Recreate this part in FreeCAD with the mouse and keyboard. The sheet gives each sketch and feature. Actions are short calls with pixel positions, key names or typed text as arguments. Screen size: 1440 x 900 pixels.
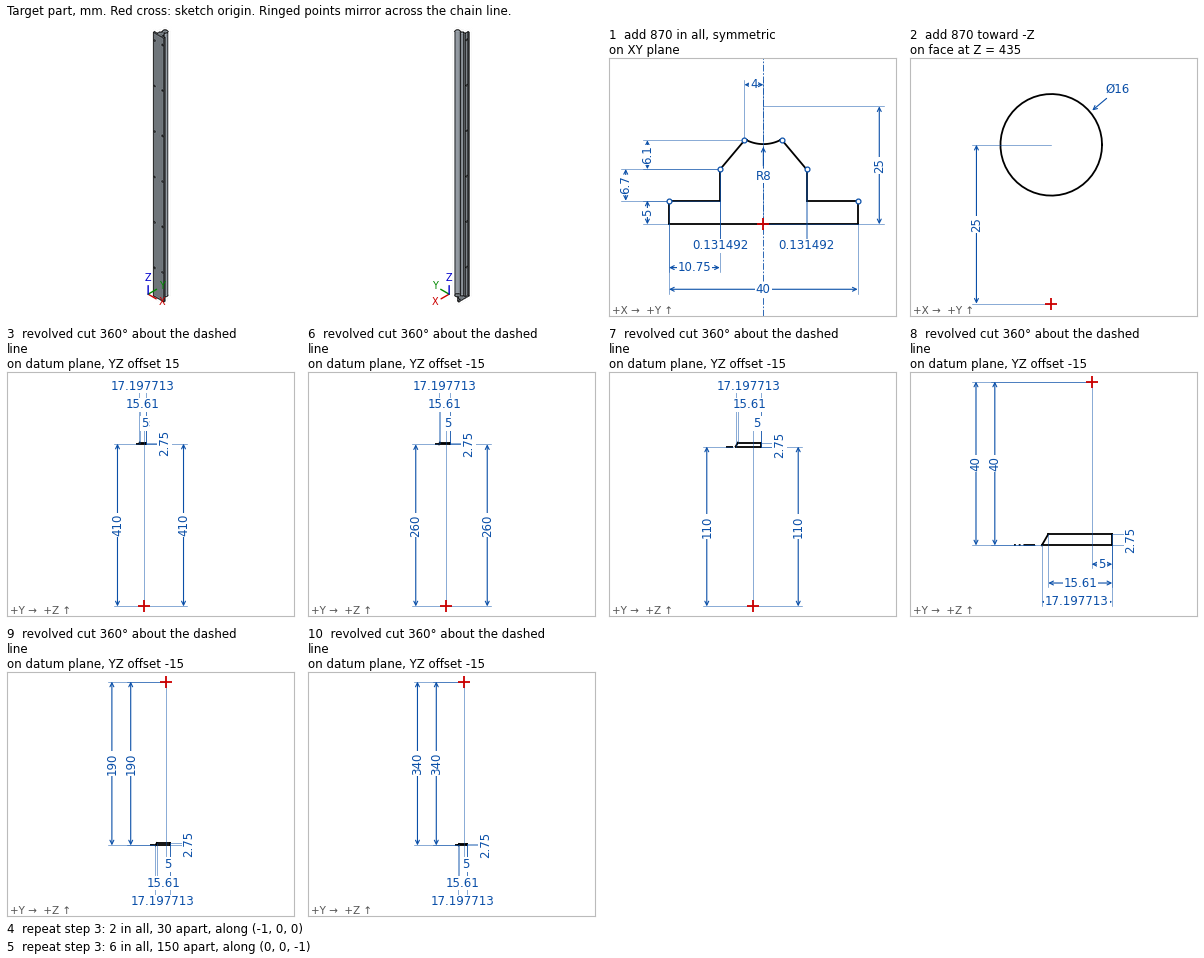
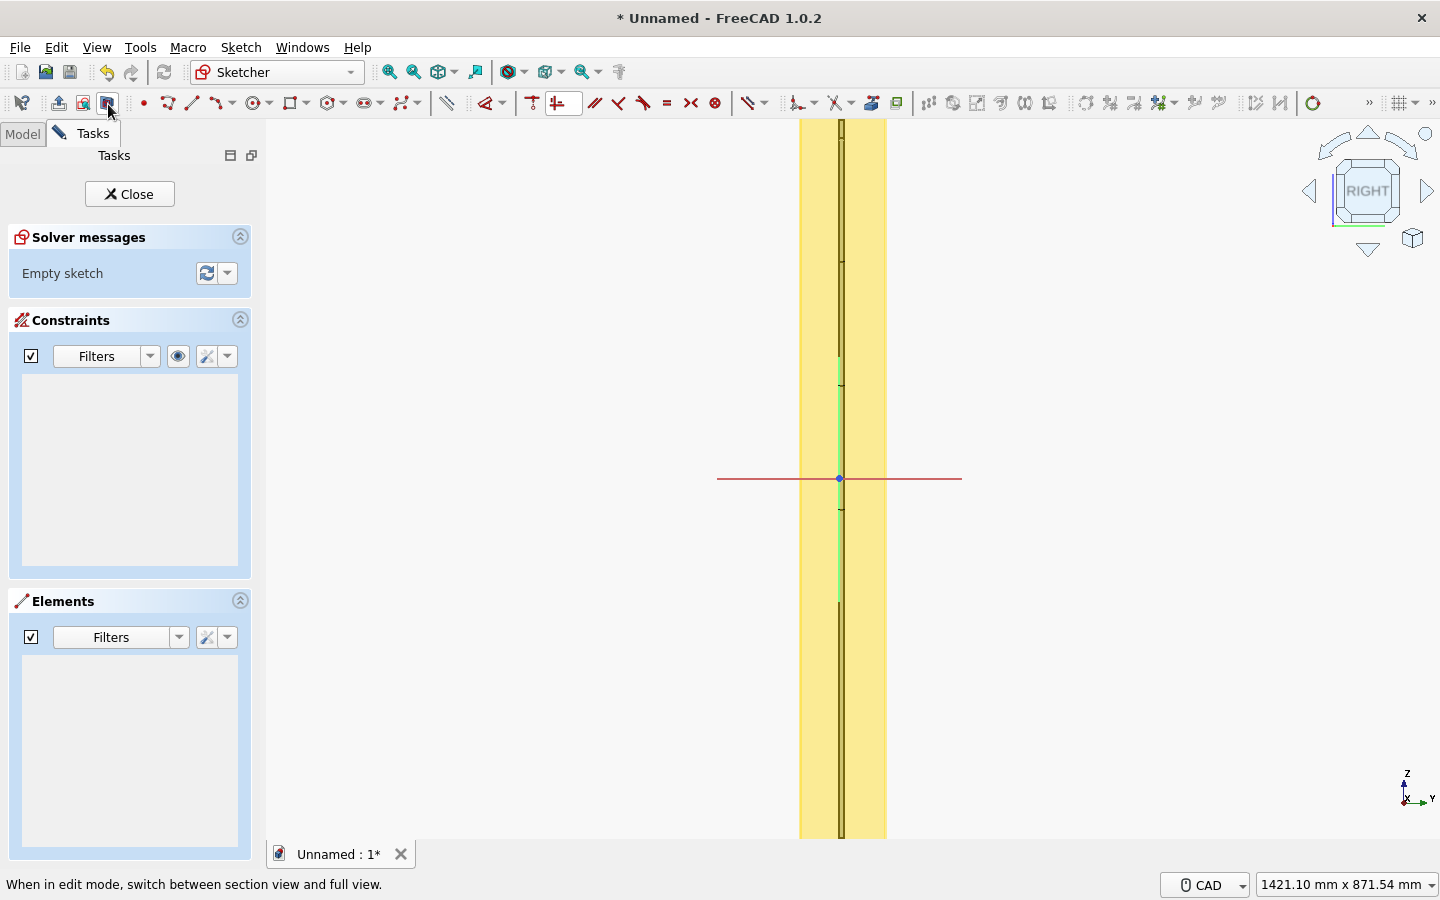
scroll(836, 643, up, 15)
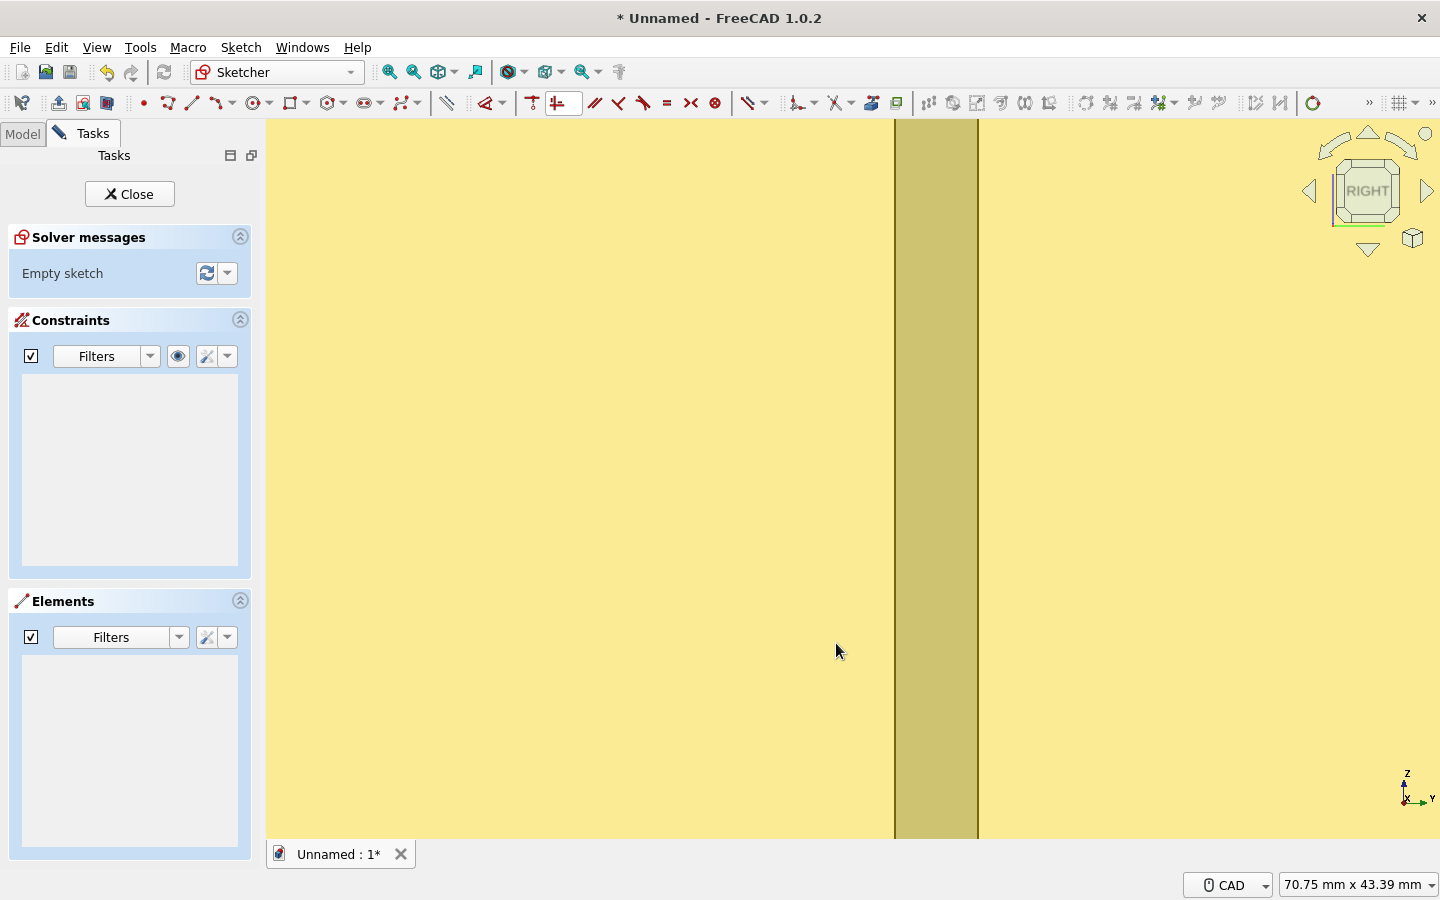
scroll(770, 448, up, 3)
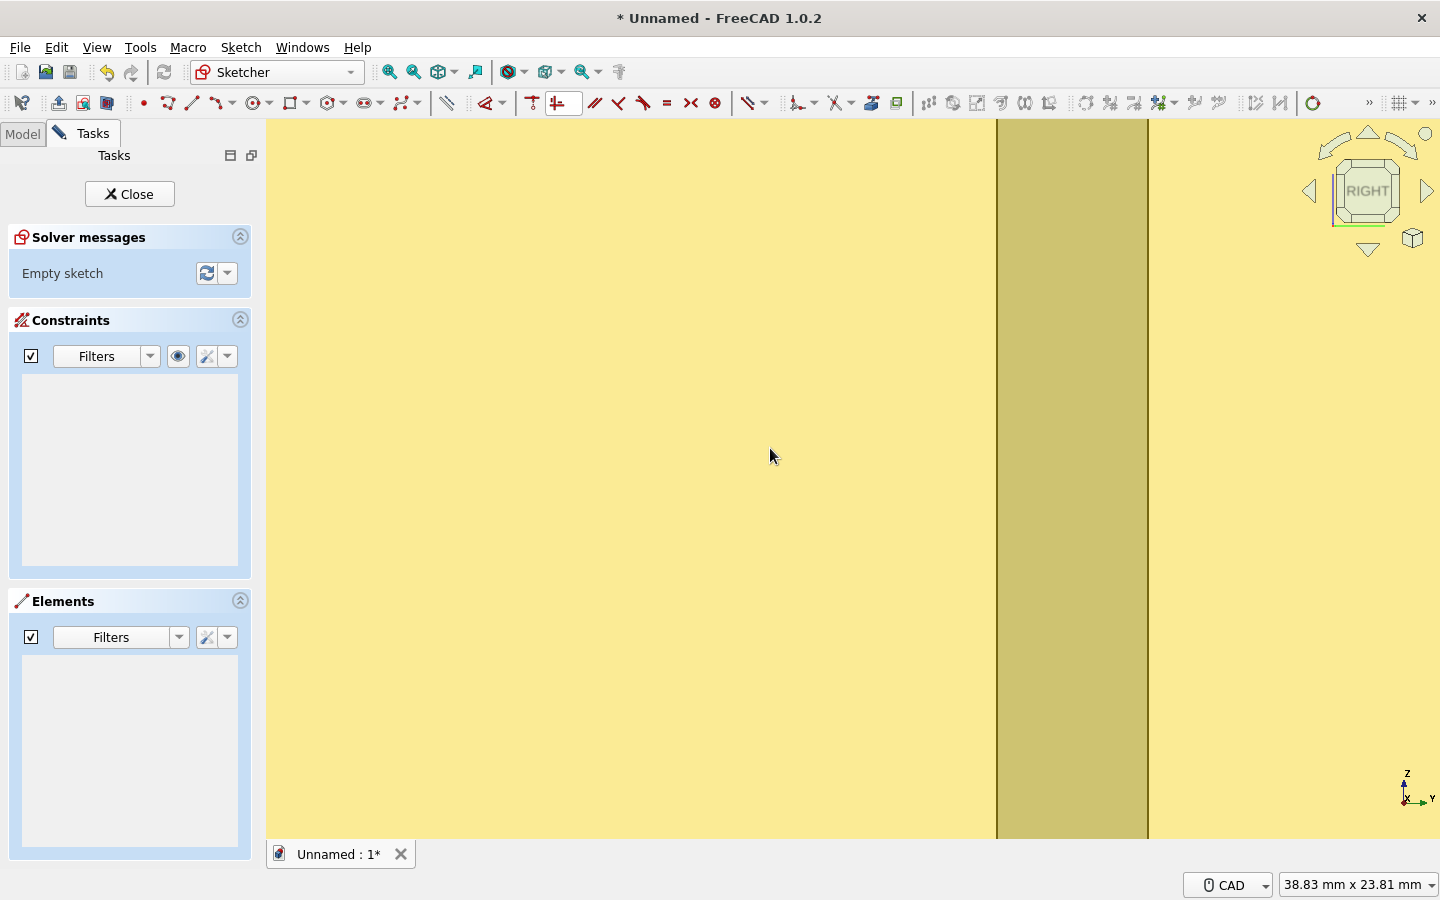
click(168, 104)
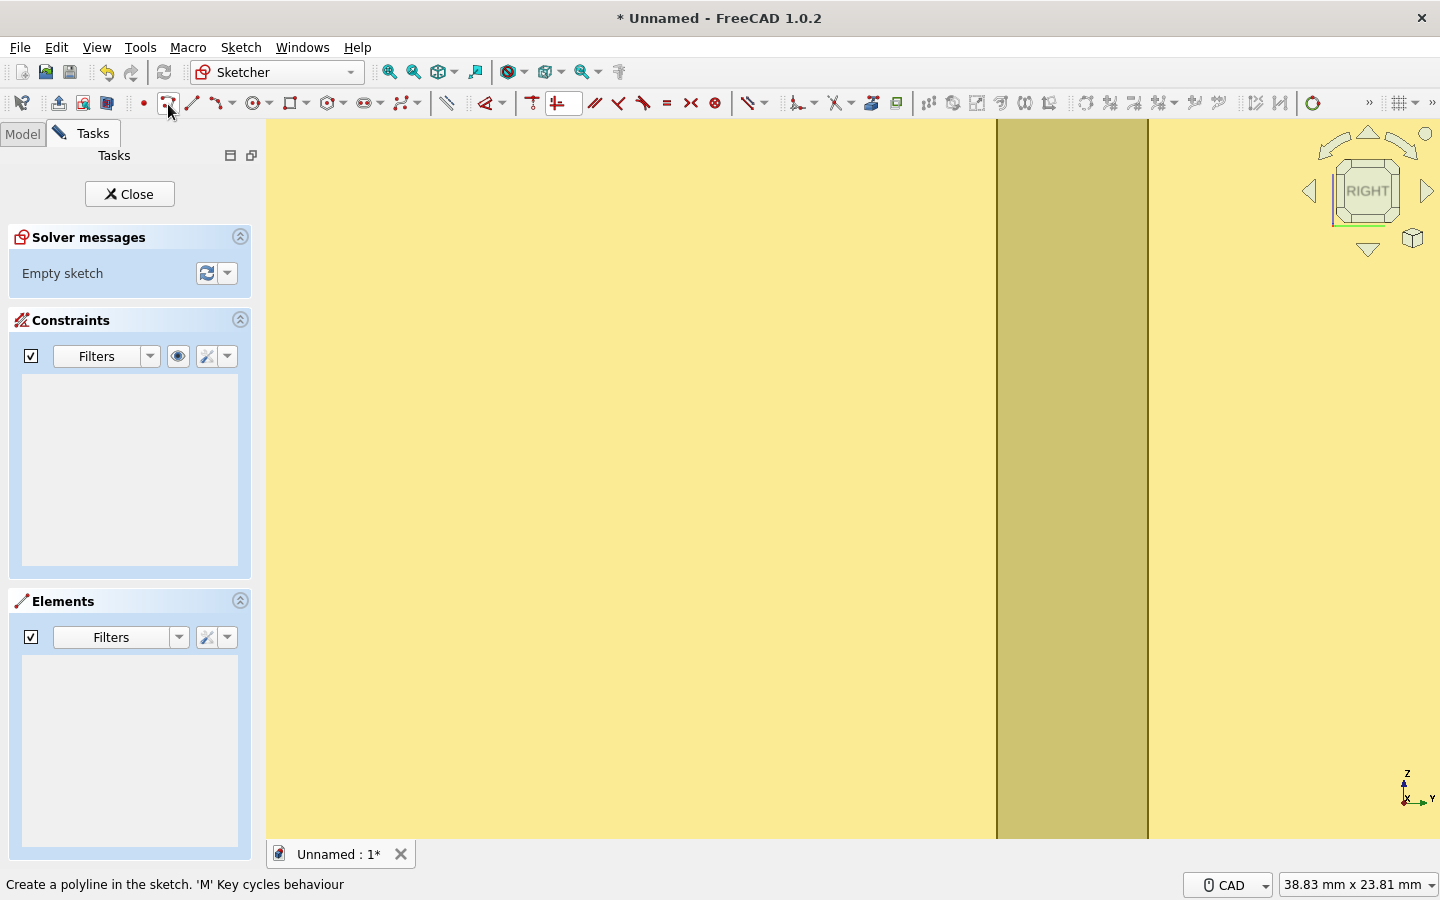
click(1148, 437)
click(676, 437)
click(628, 520)
click(1148, 520)
click(1148, 438)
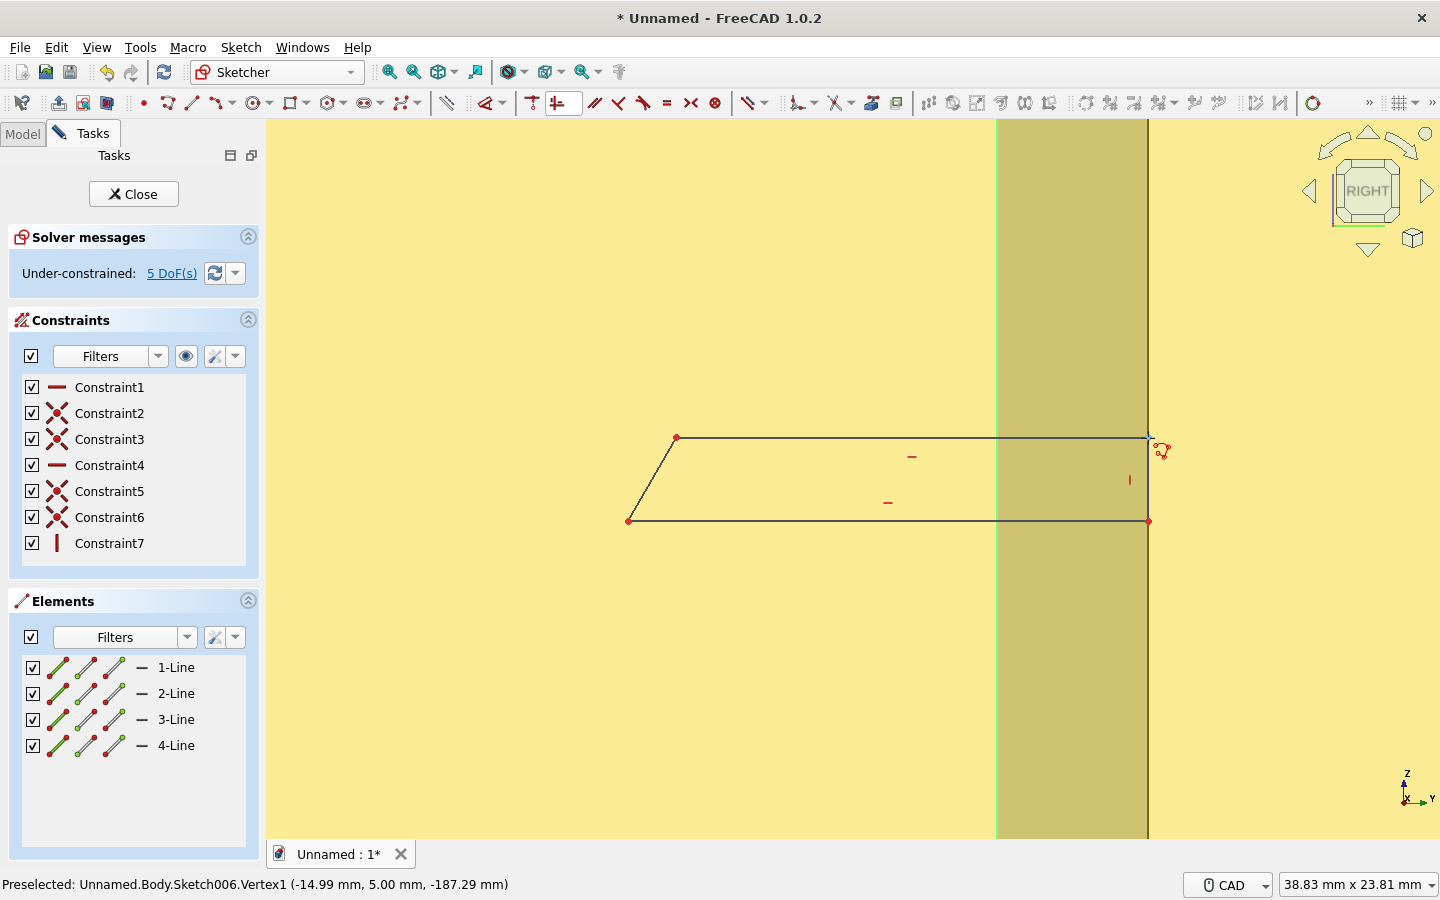
click(192, 104)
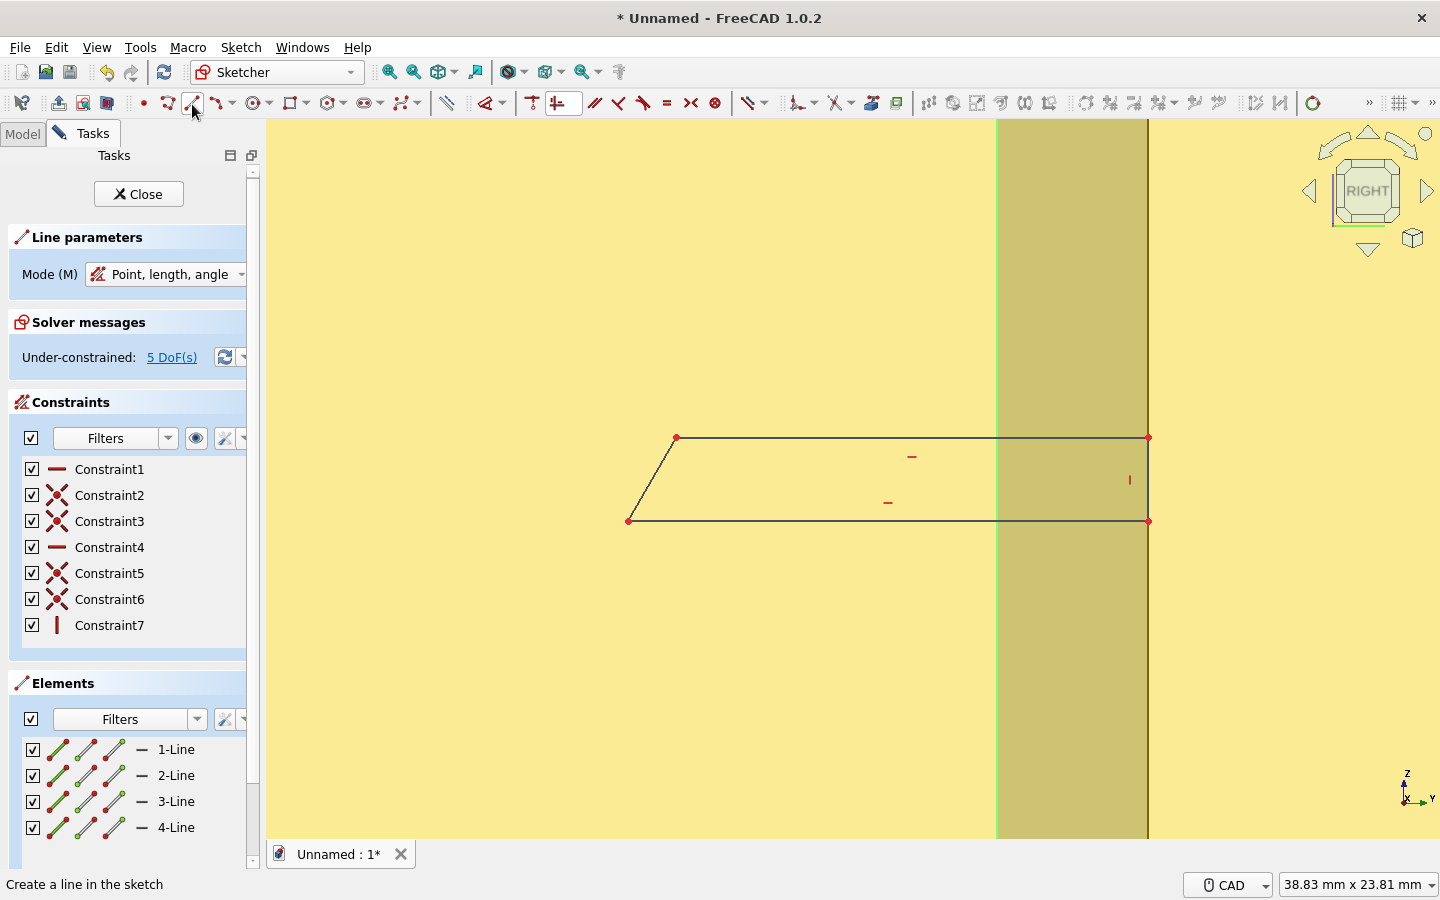
click(576, 520)
click(420, 520)
key(Escape)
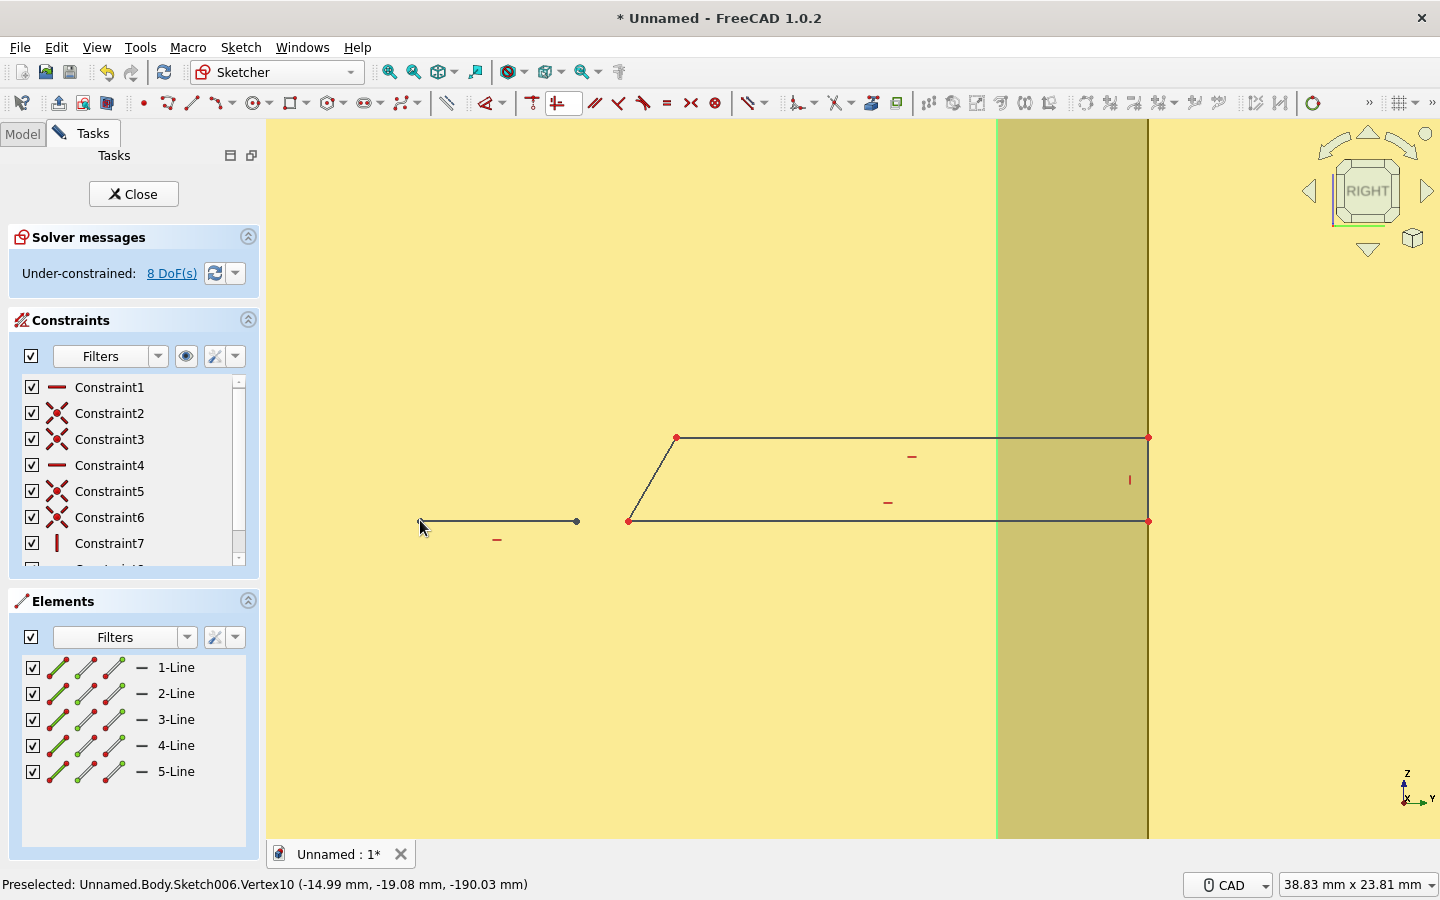
click(529, 521)